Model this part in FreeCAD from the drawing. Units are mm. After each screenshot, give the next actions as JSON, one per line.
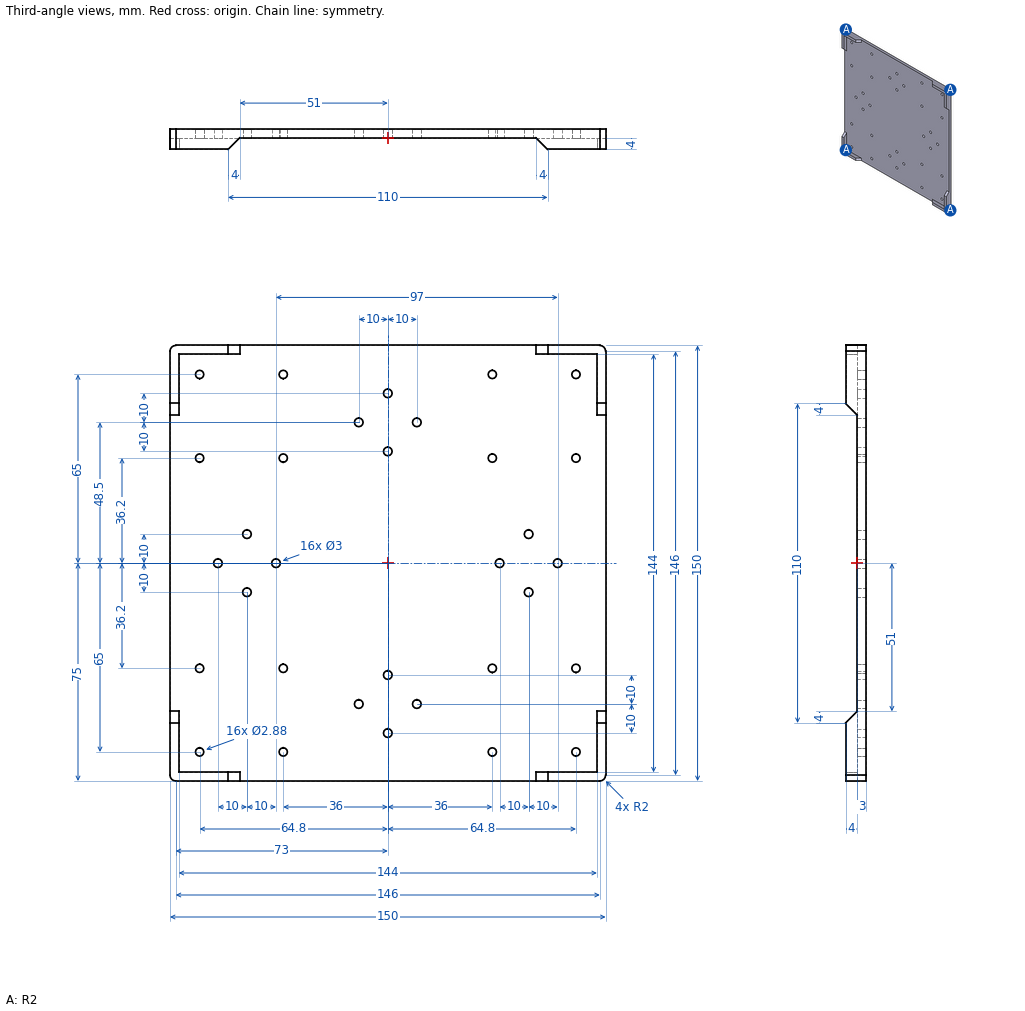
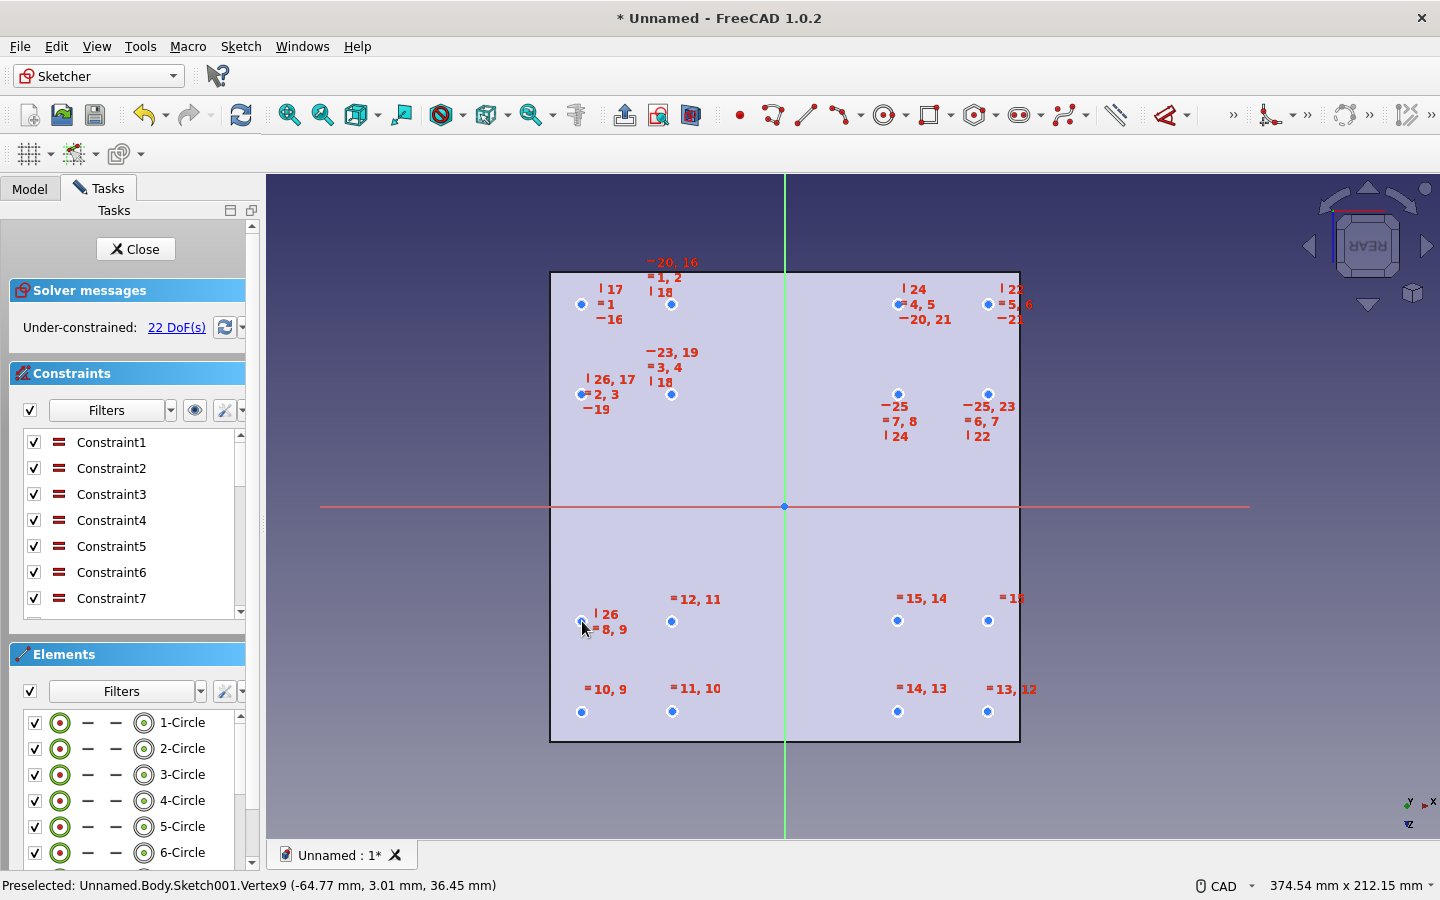
{"action": "left_click", "coordinate": [581, 621]}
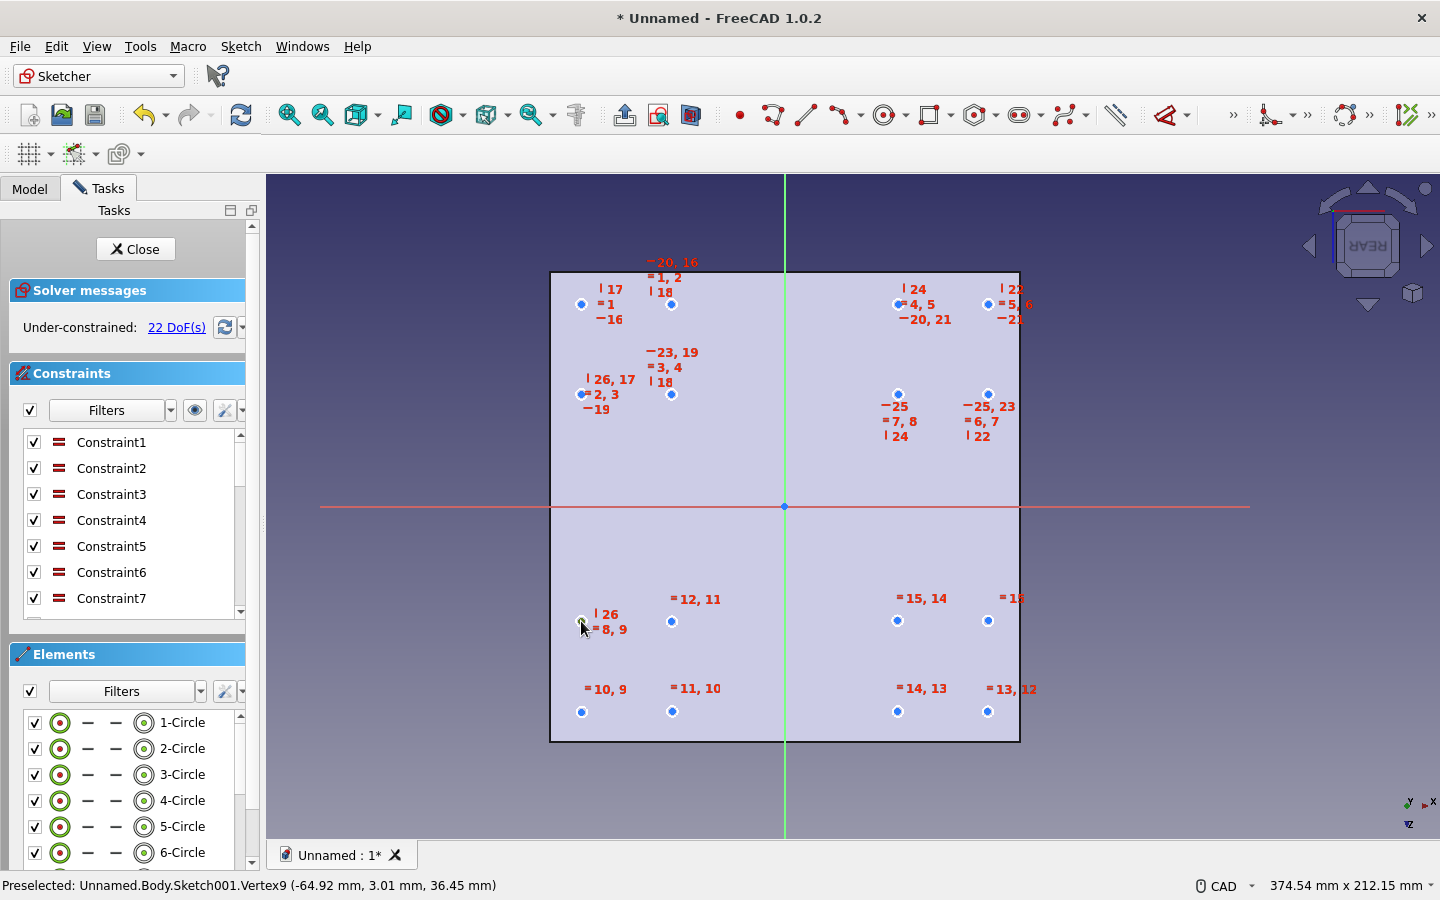
{"action": "left_click", "coordinate": [582, 712]}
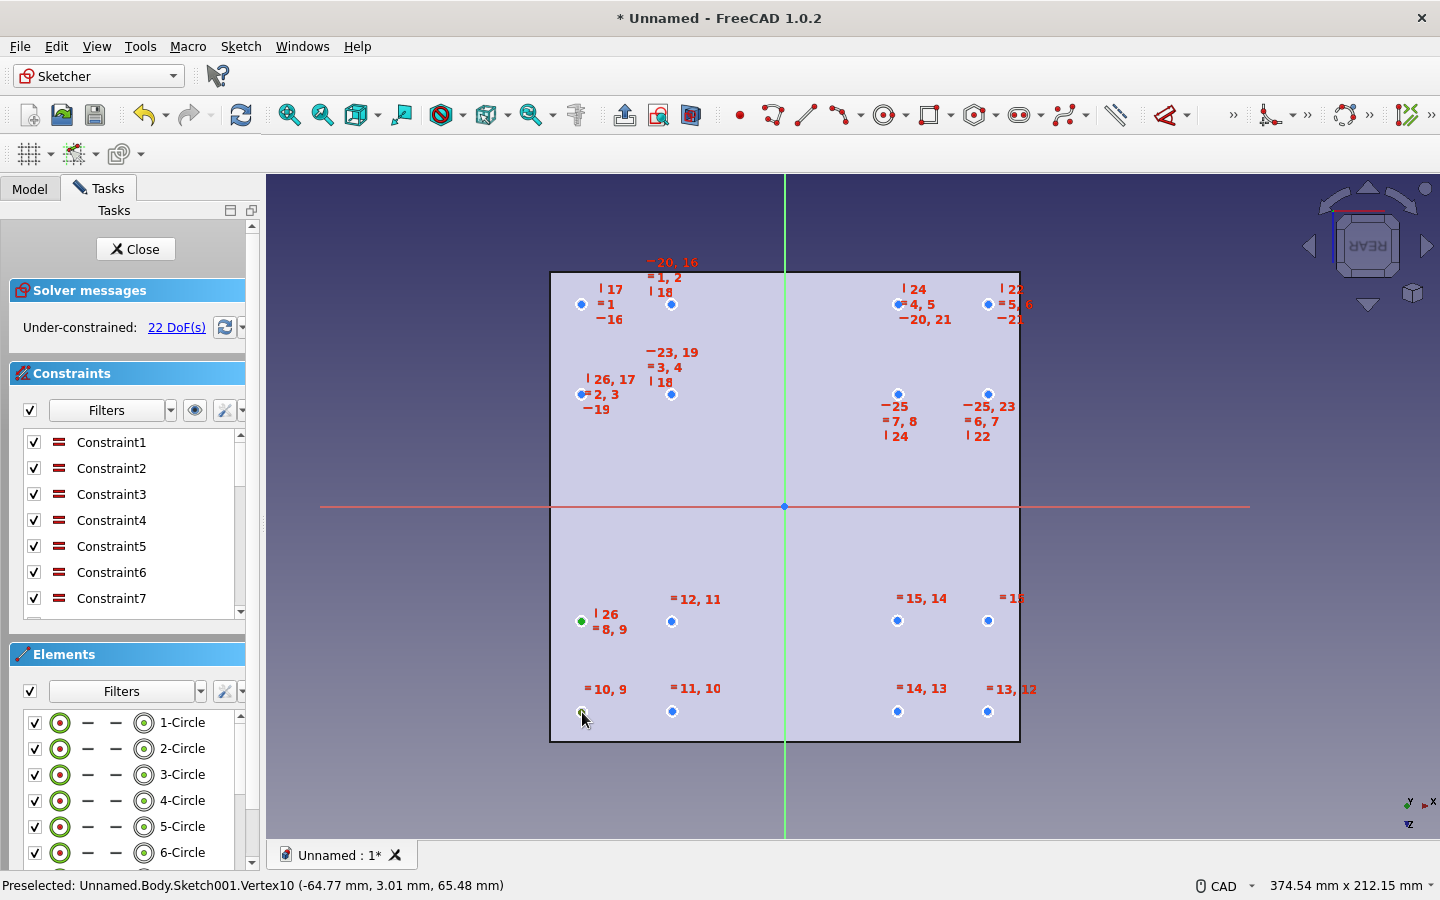
{"action": "key", "text": "v"}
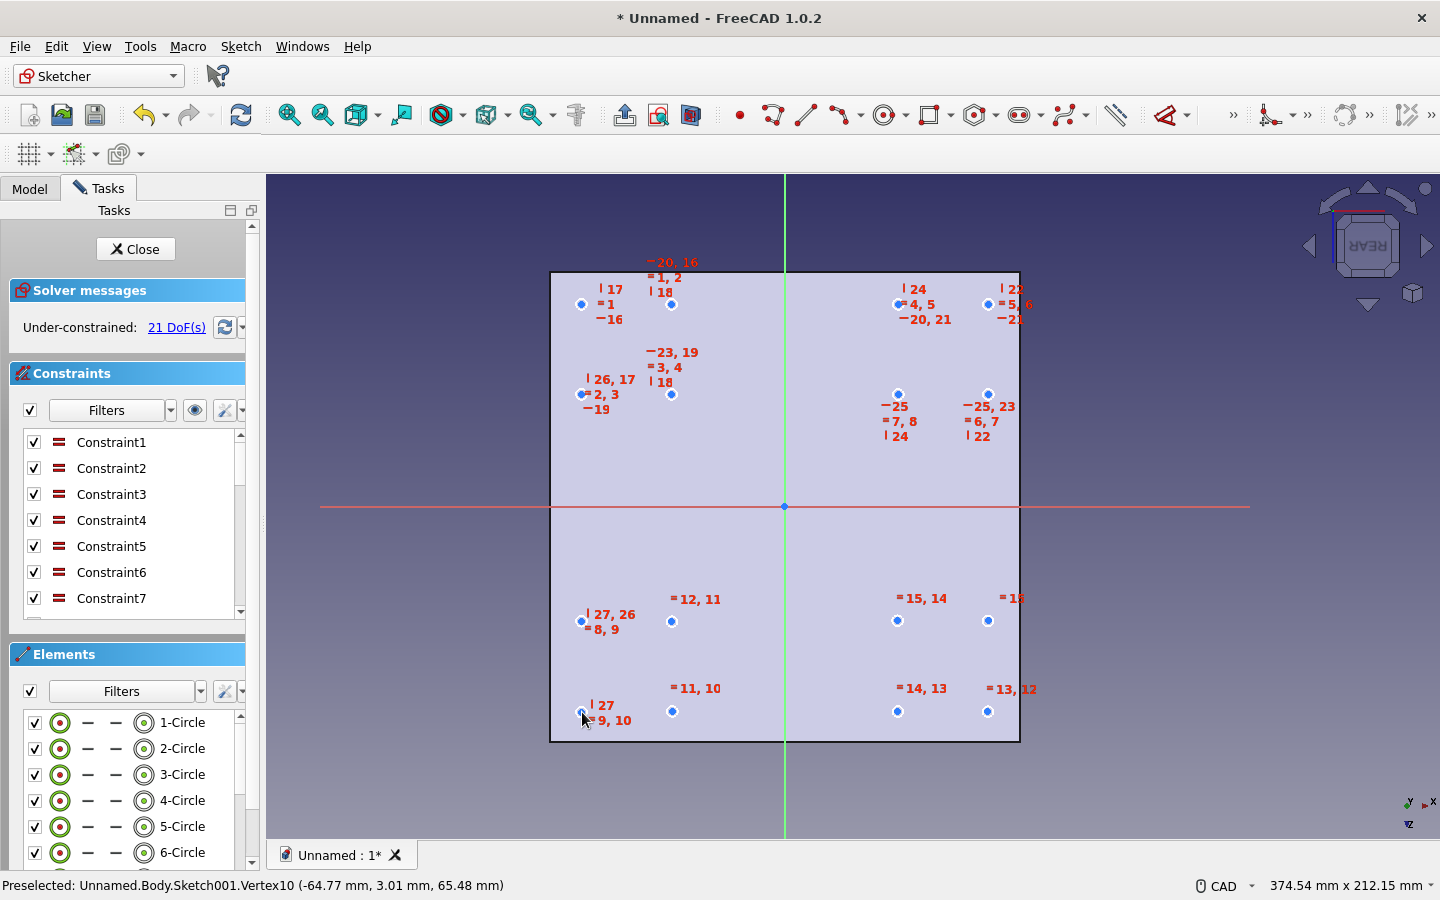
{"action": "left_click", "coordinate": [672, 394]}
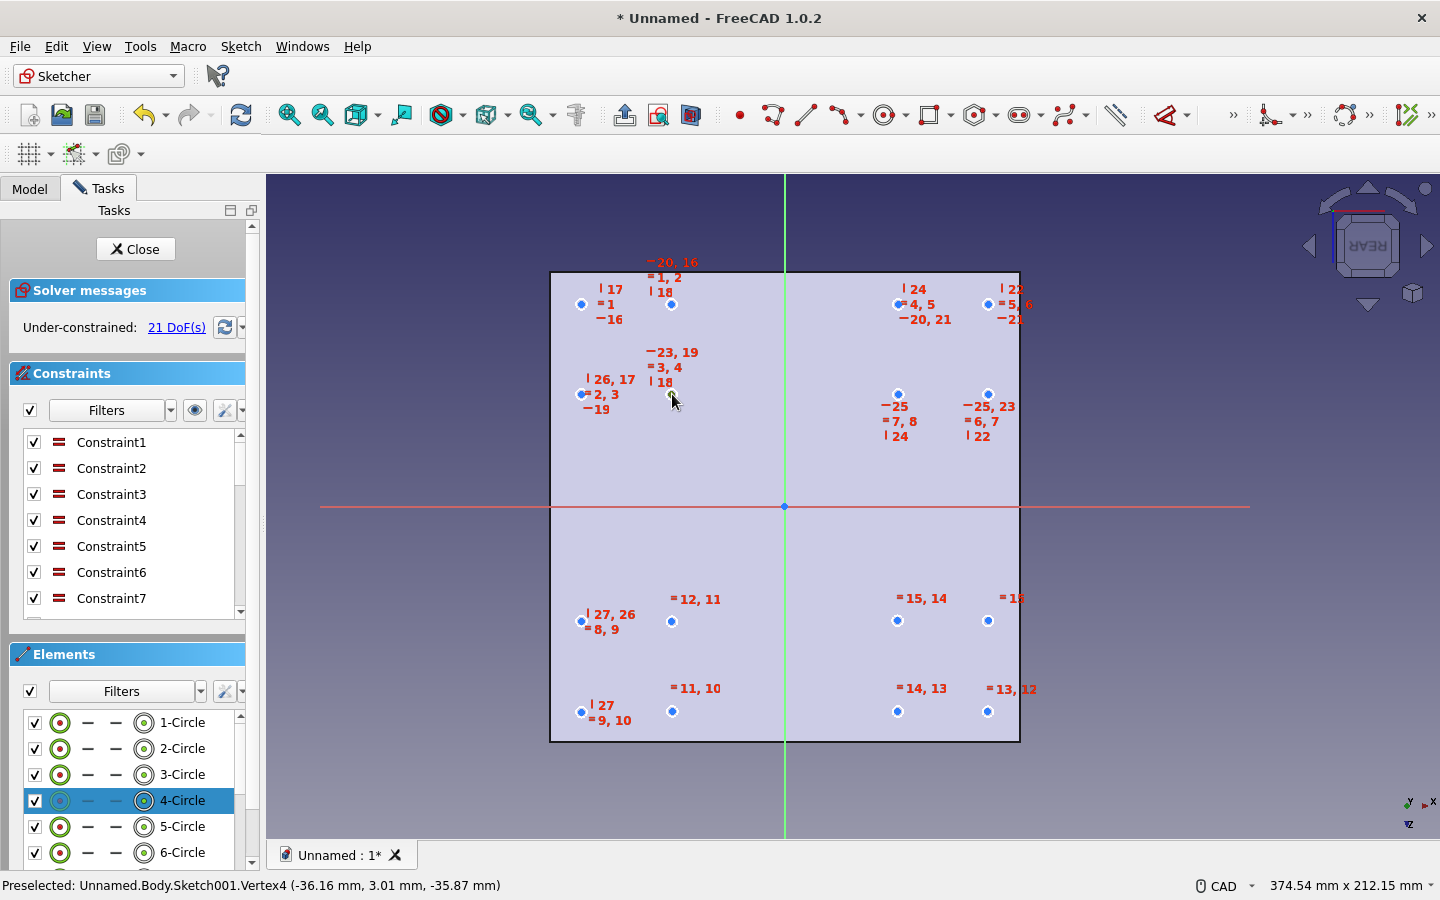
{"action": "left_click", "coordinate": [672, 711]}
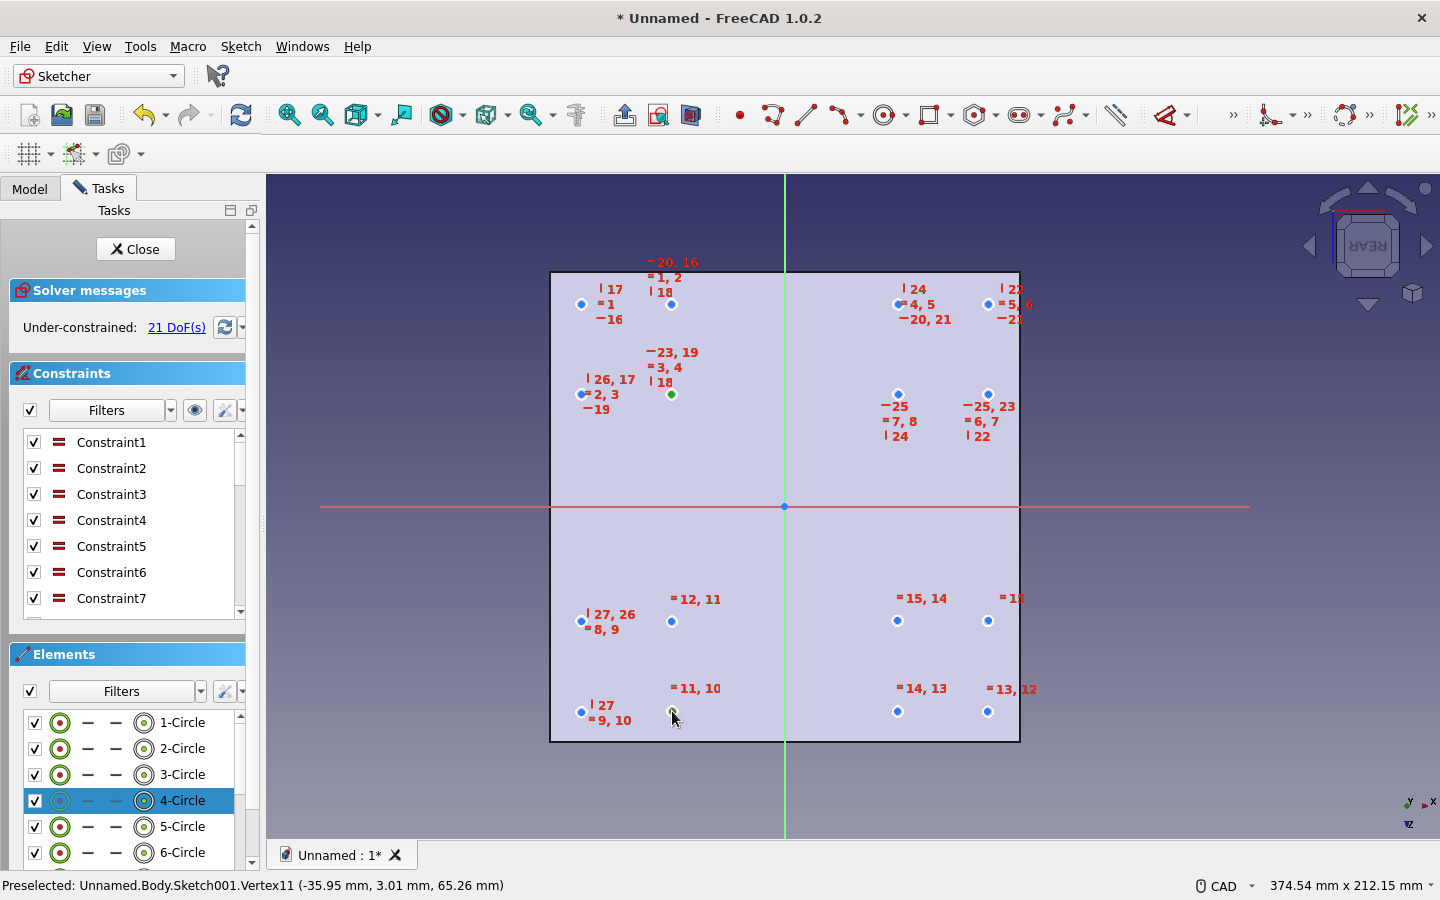
{"action": "key", "text": "v"}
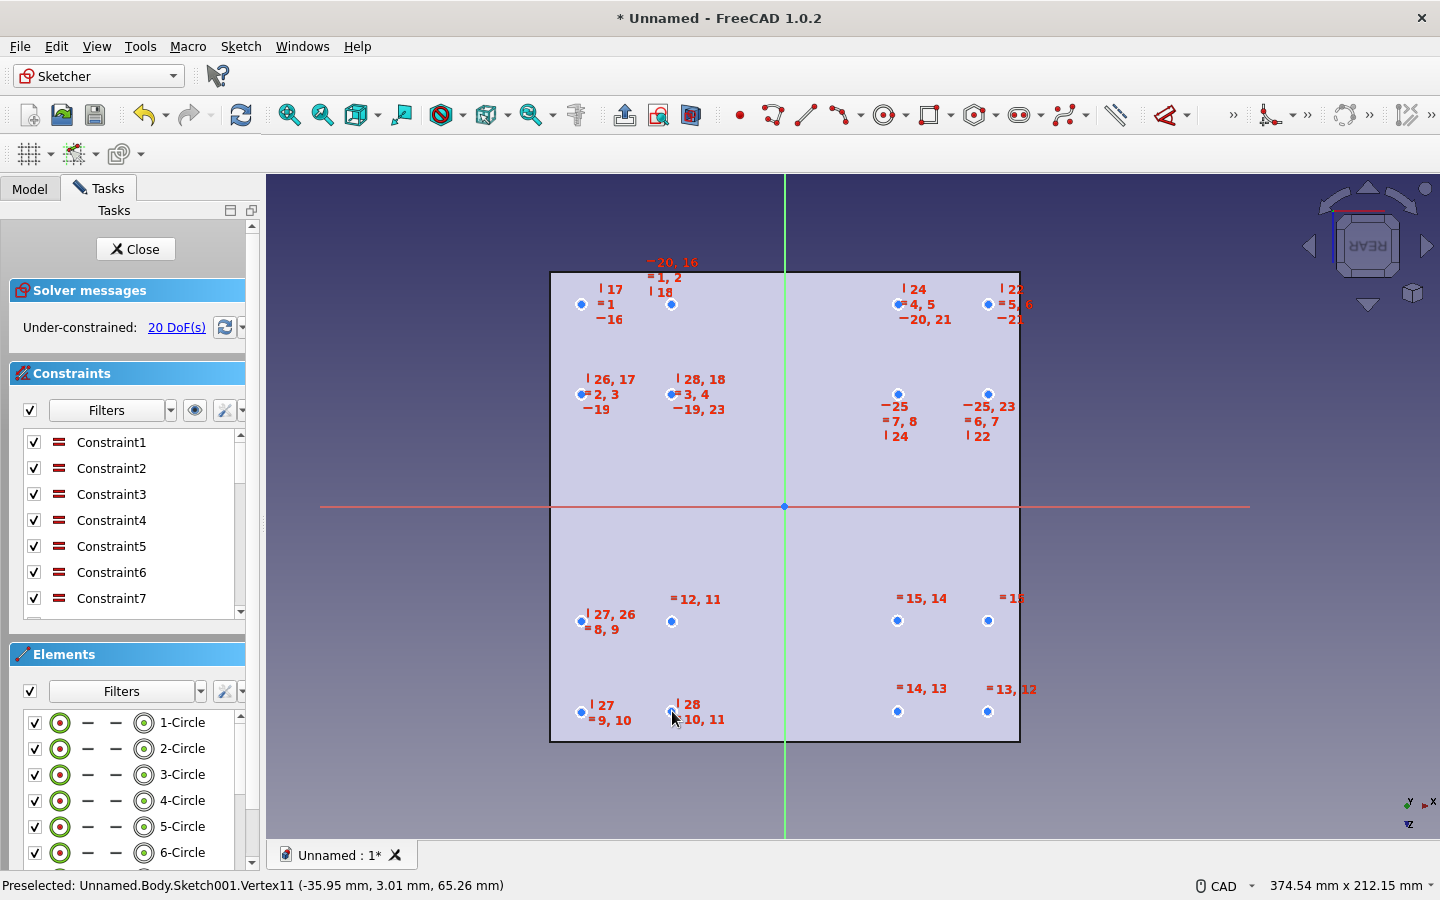
{"action": "left_click", "coordinate": [581, 712]}